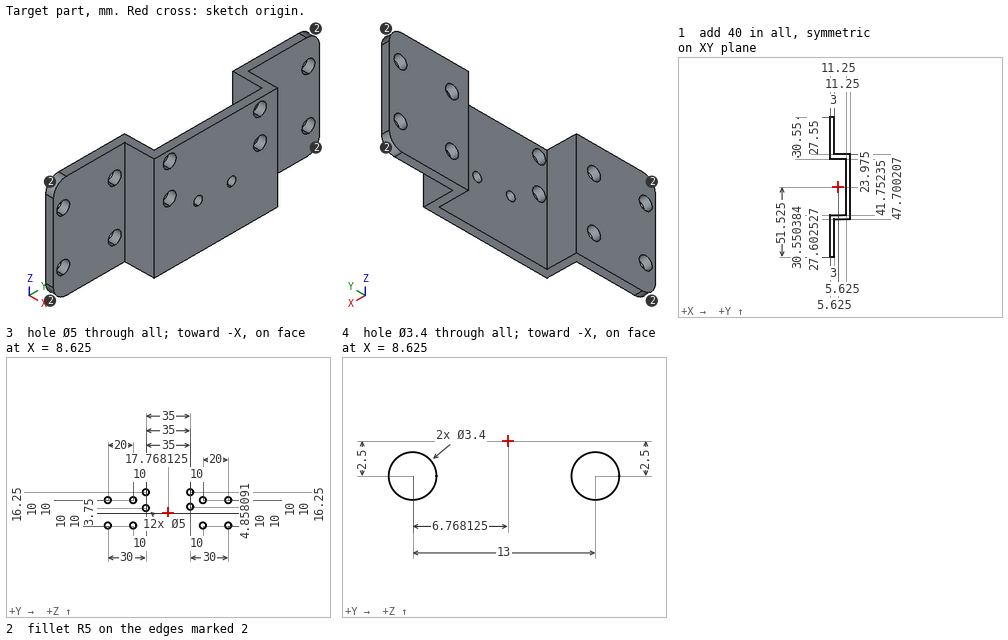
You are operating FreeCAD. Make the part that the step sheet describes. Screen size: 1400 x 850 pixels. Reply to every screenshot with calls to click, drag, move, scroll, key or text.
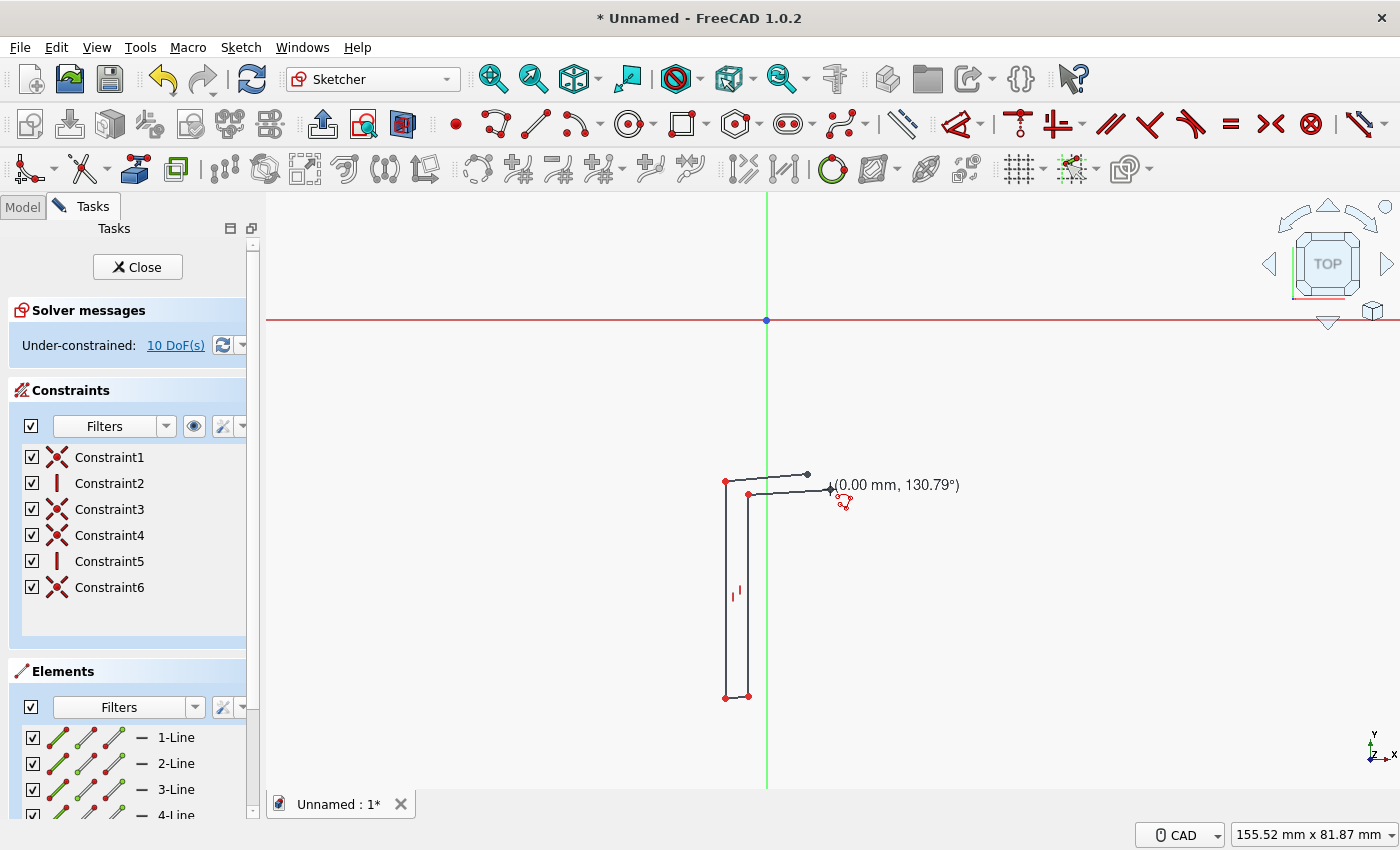
scroll(748, 698, down, 3)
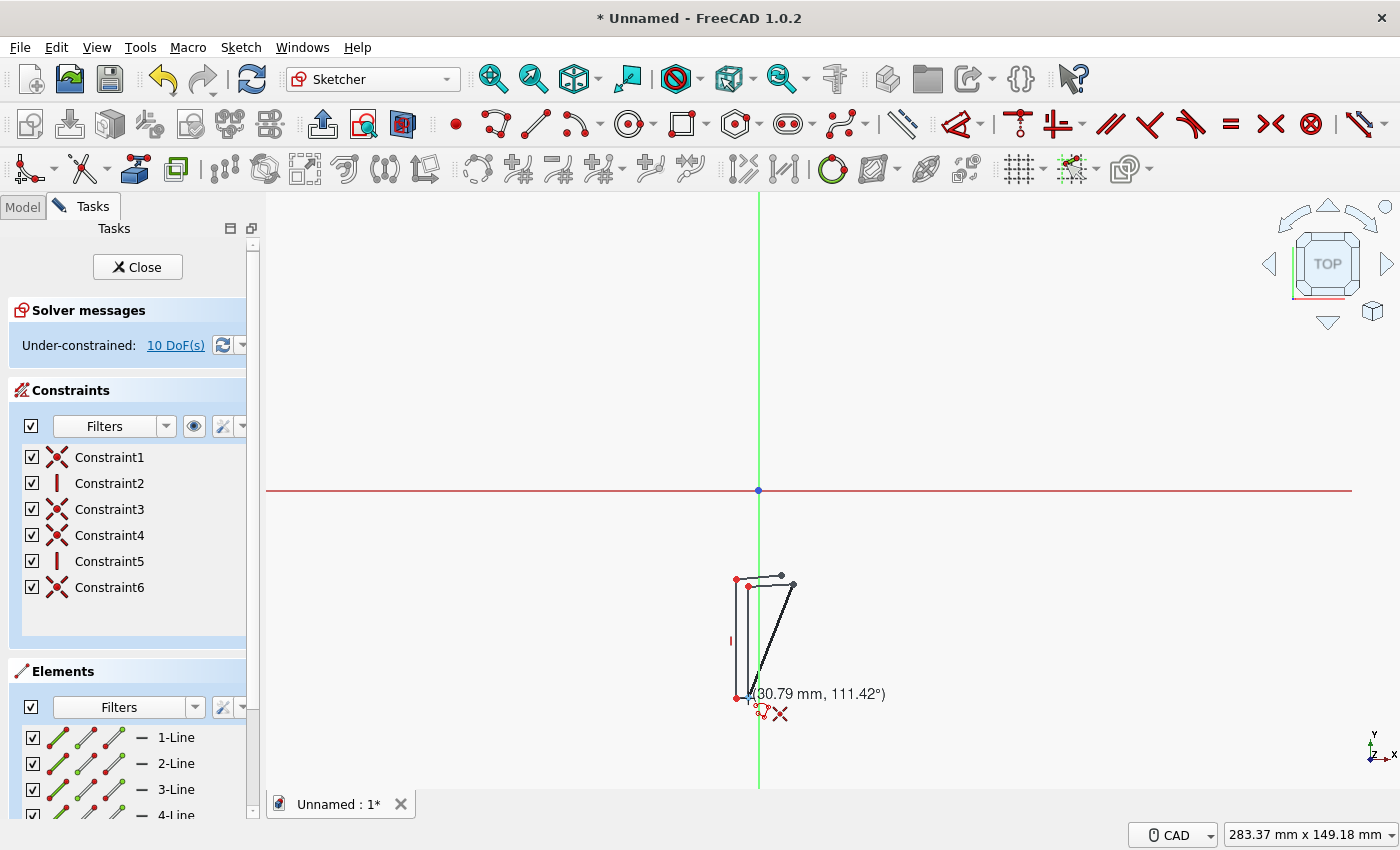
click(793, 395)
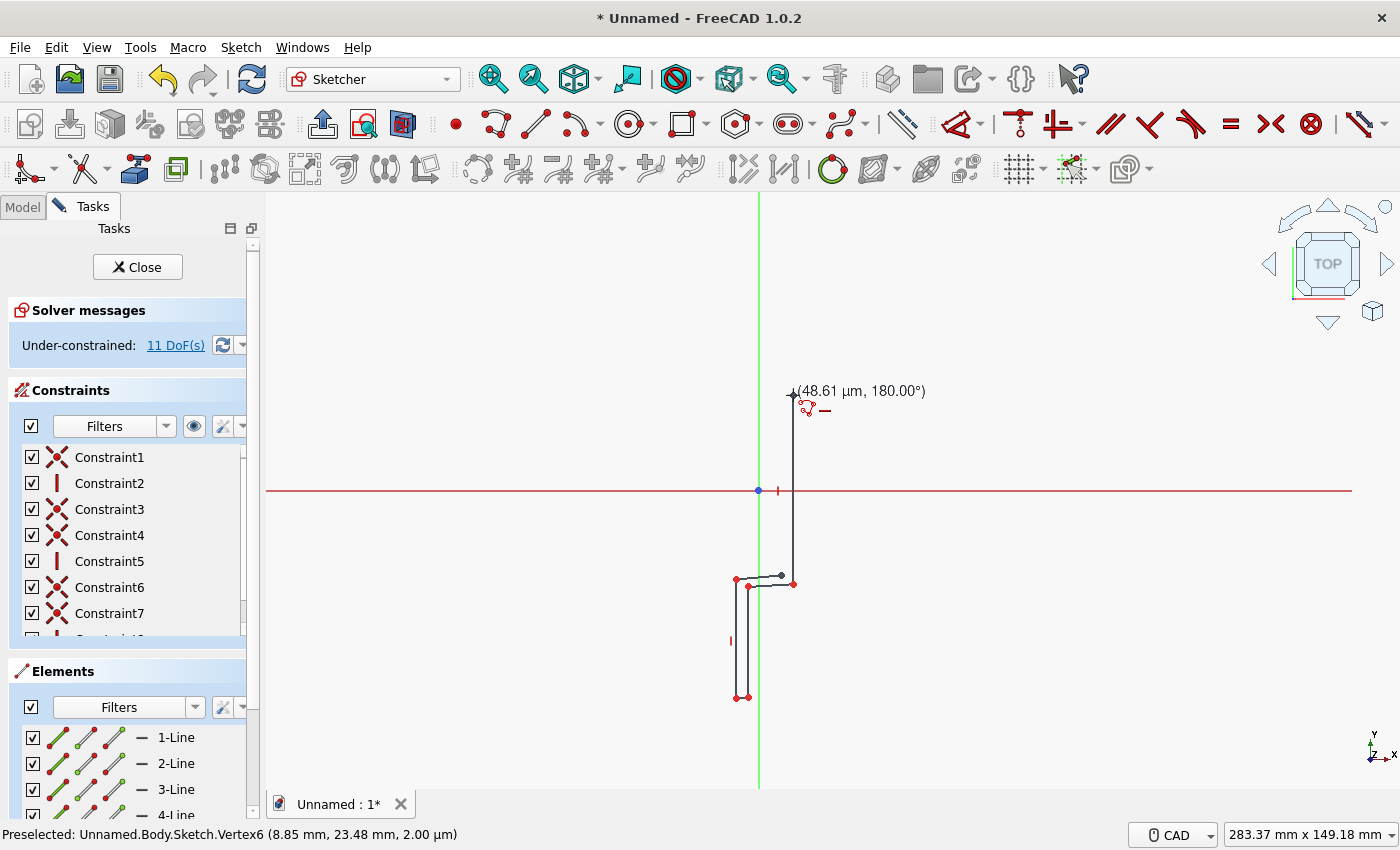
scroll(748, 395, up, 3)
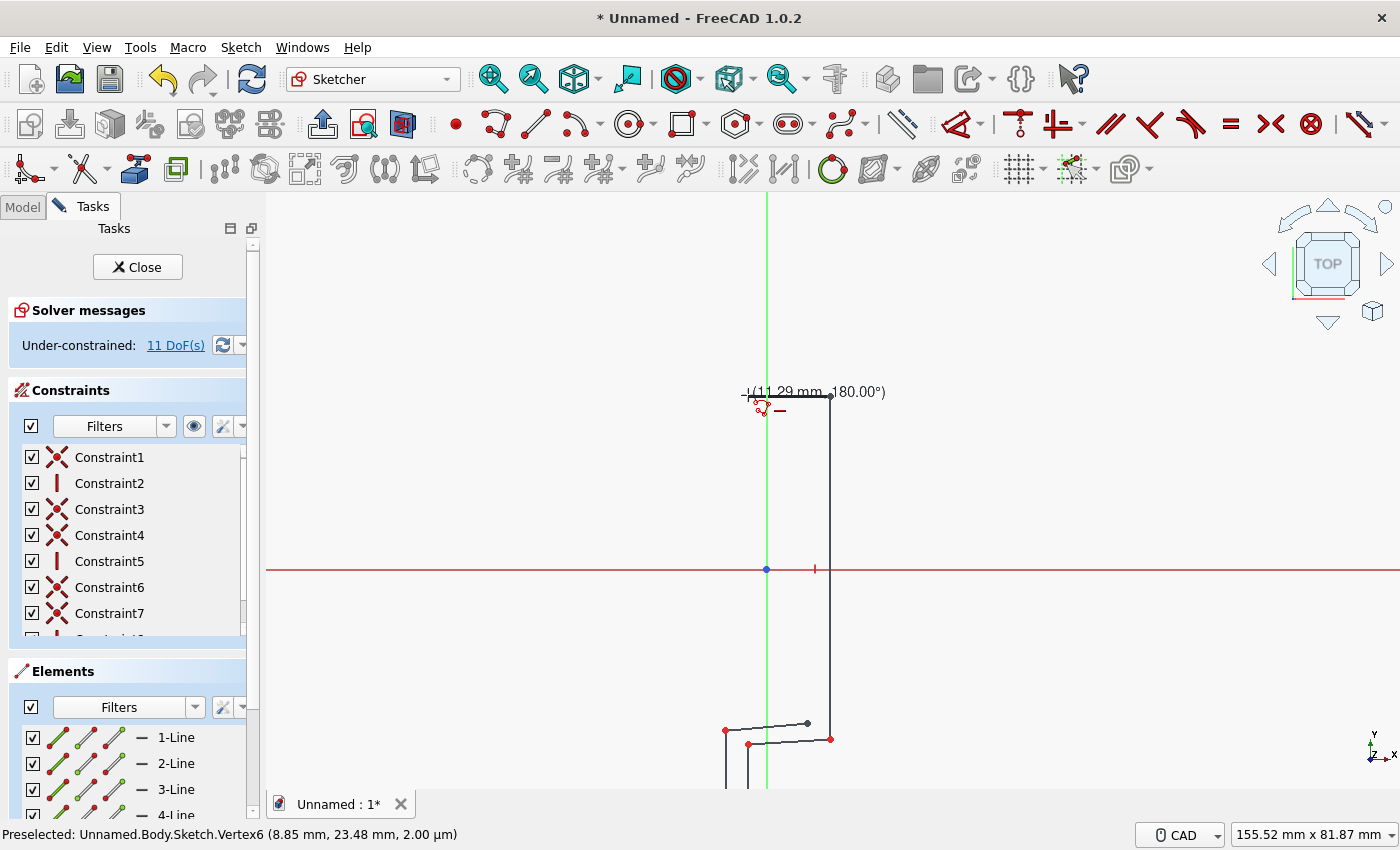
click(748, 395)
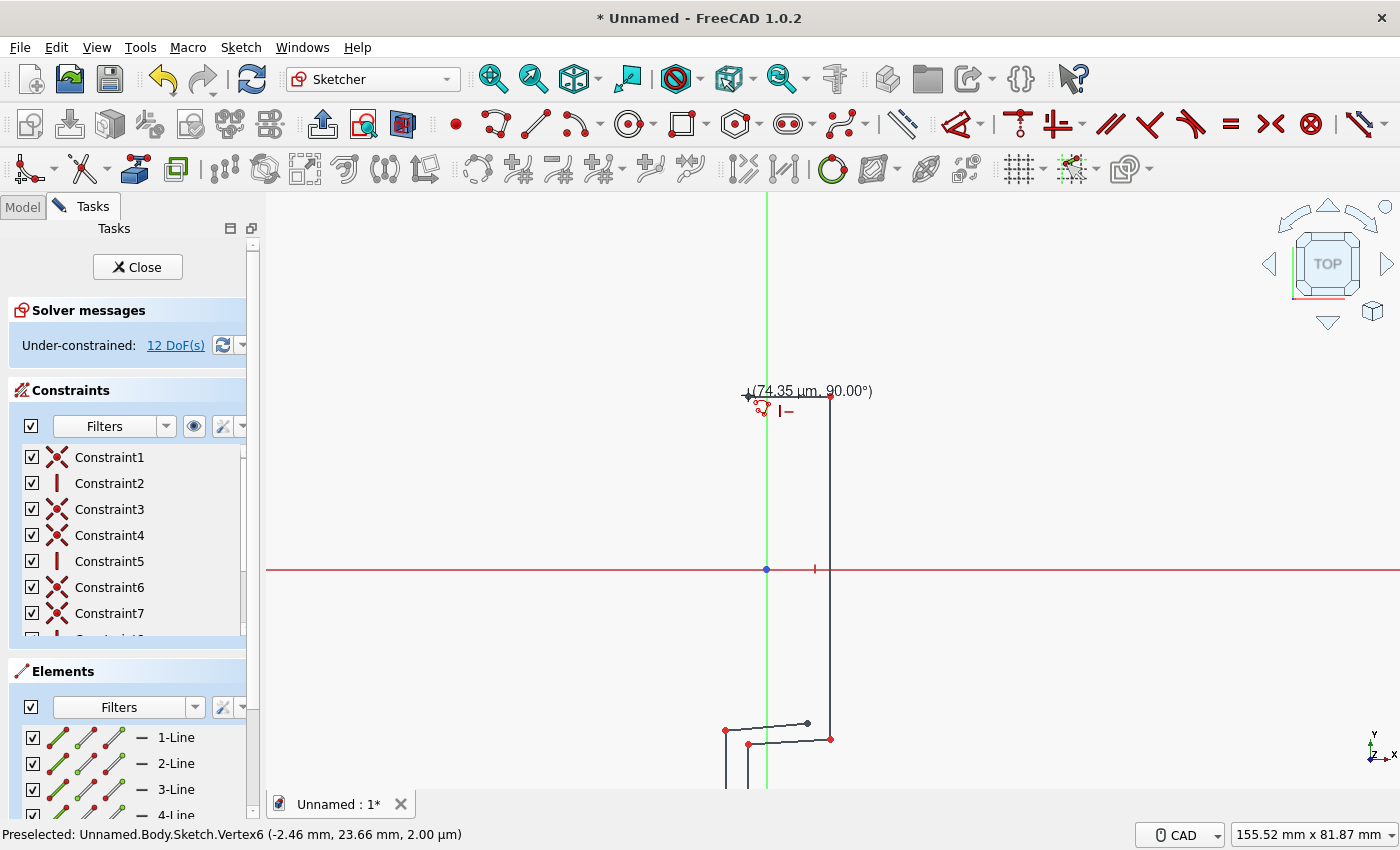
scroll(748, 394, down, 3)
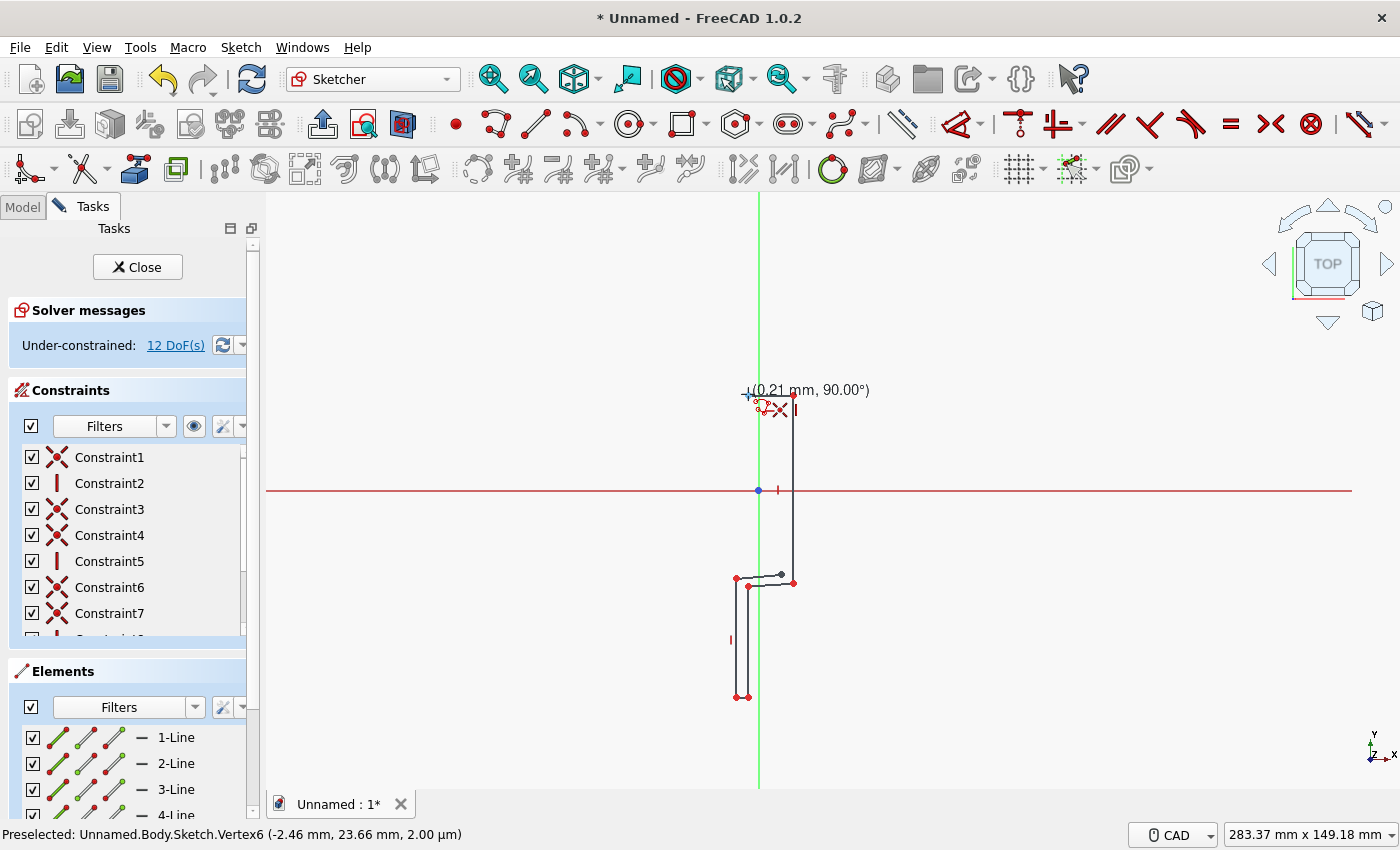
scroll(748, 284, up, 3)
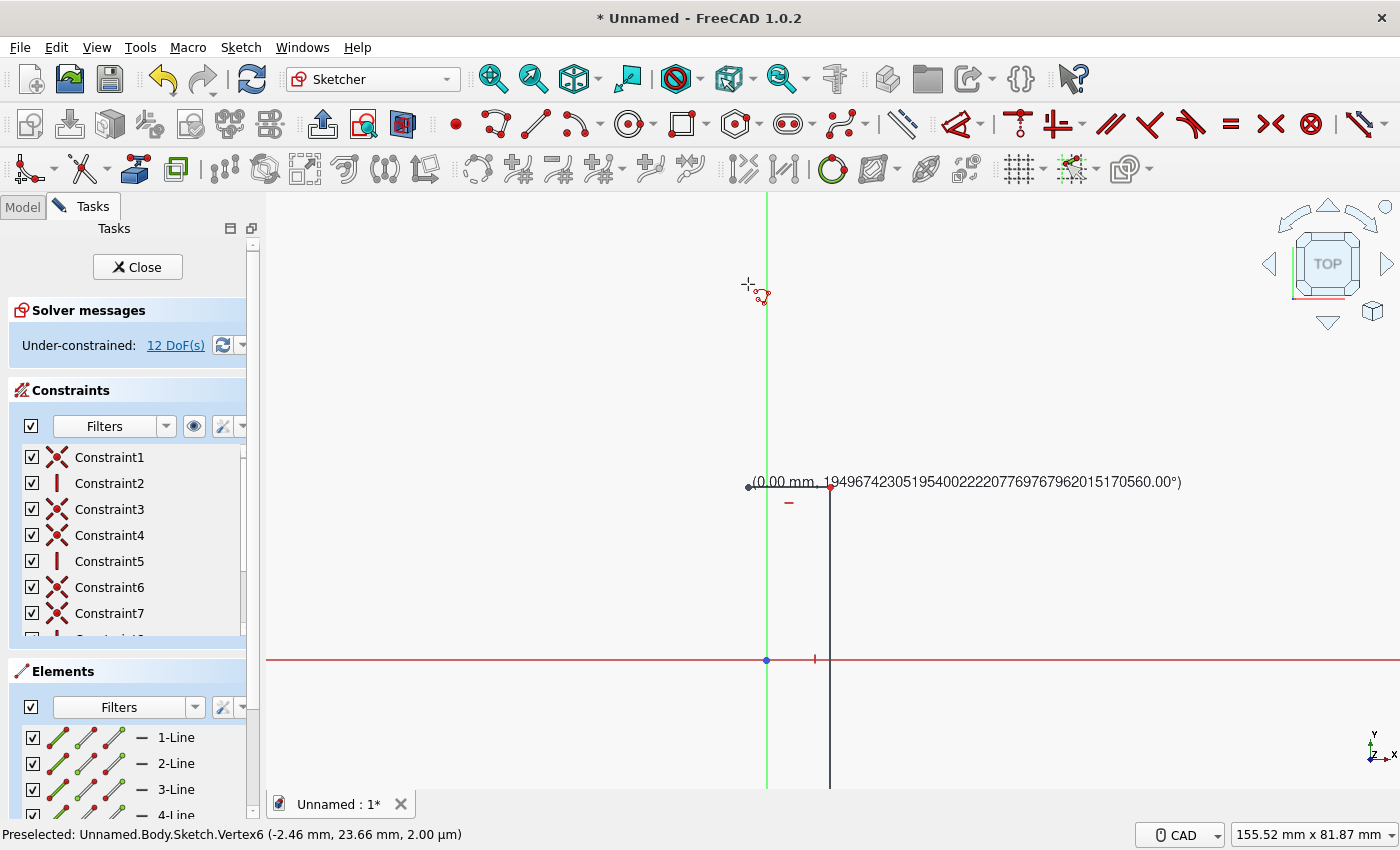
click(748, 284)
click(726, 284)
click(726, 507)
click(808, 507)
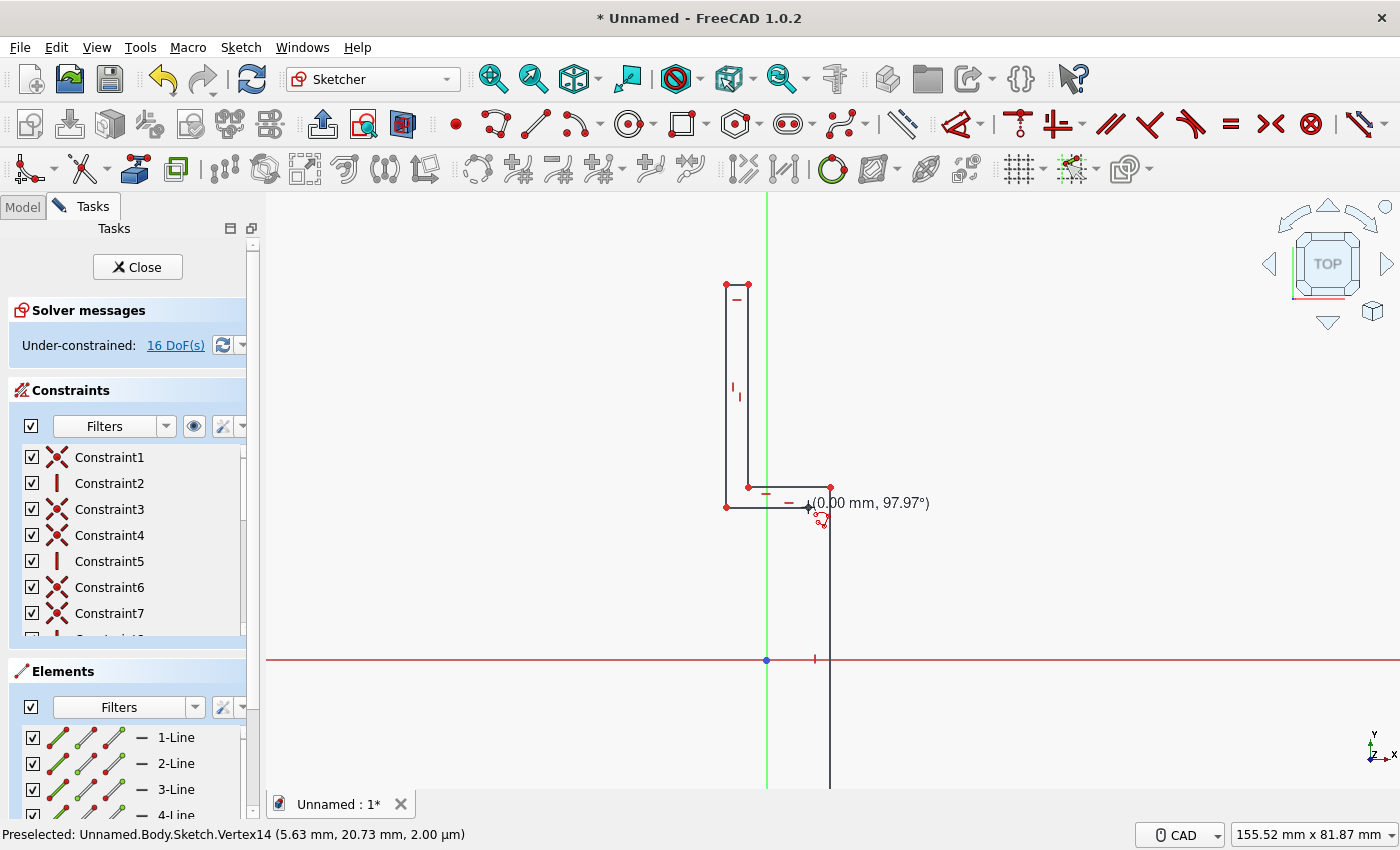
scroll(748, 284, down, 3)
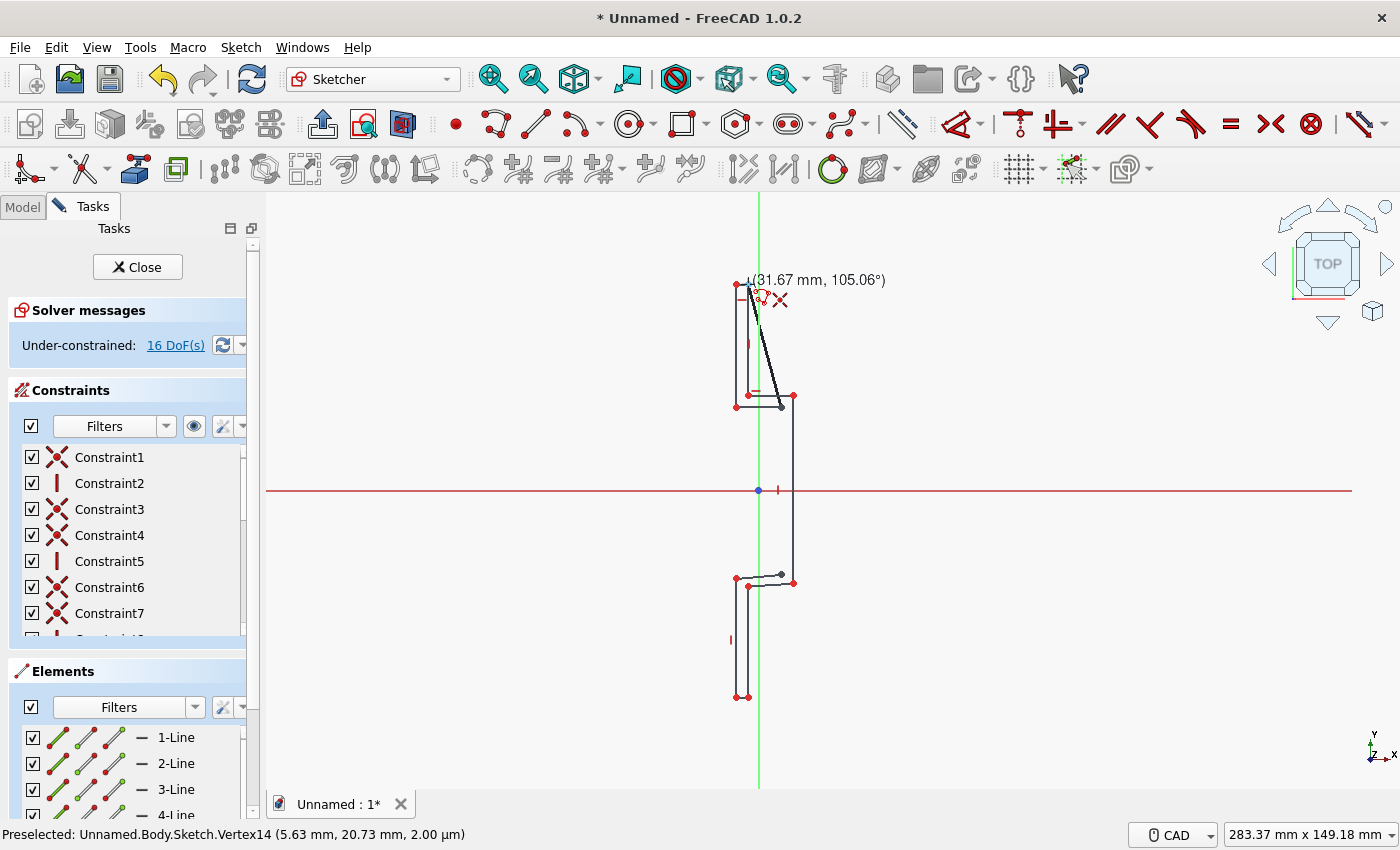
scroll(781, 574, up, 2)